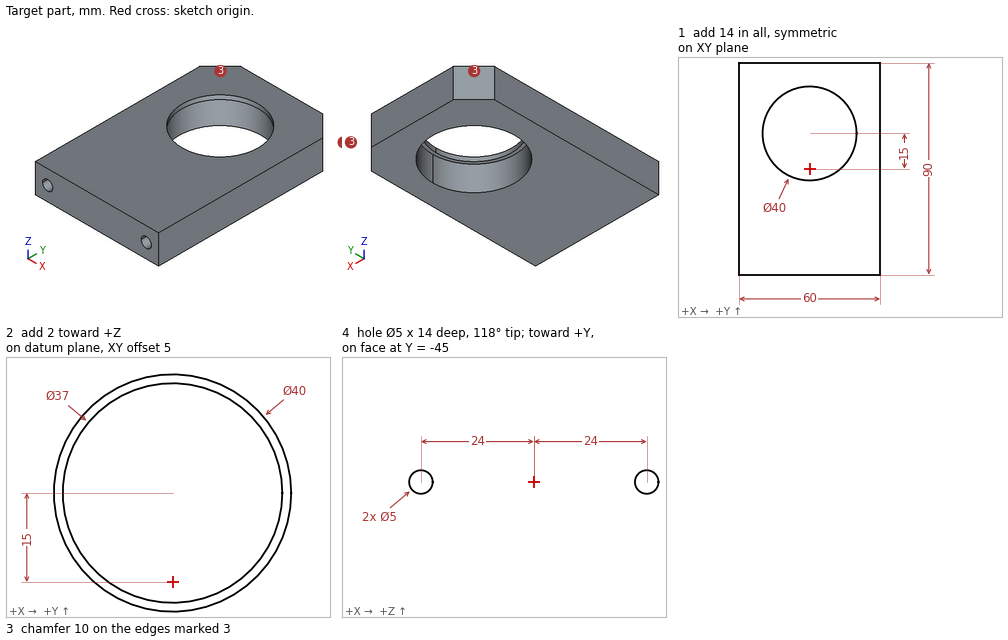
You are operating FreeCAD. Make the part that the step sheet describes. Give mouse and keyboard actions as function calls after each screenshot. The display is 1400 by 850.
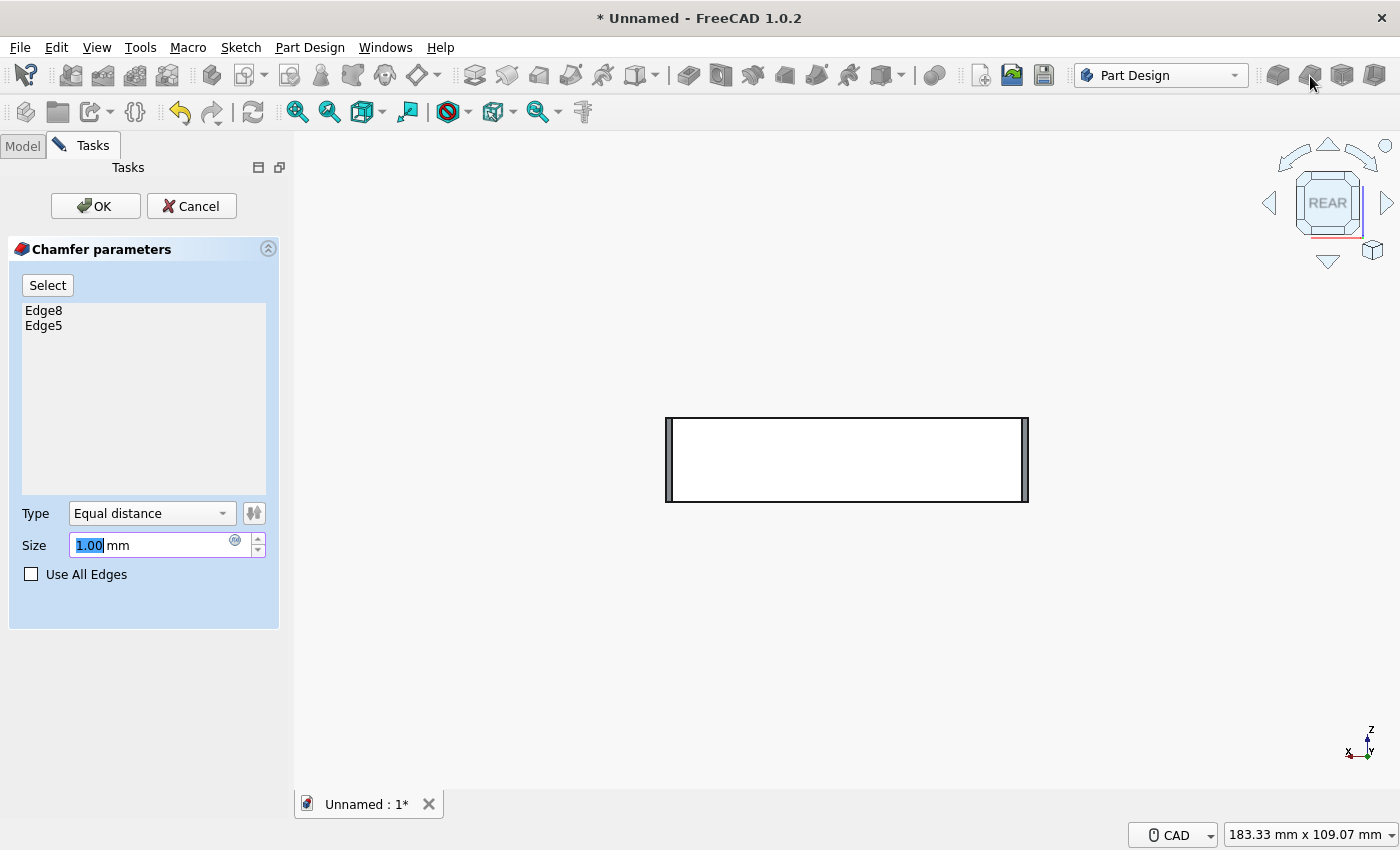
text(10)
key(Tab)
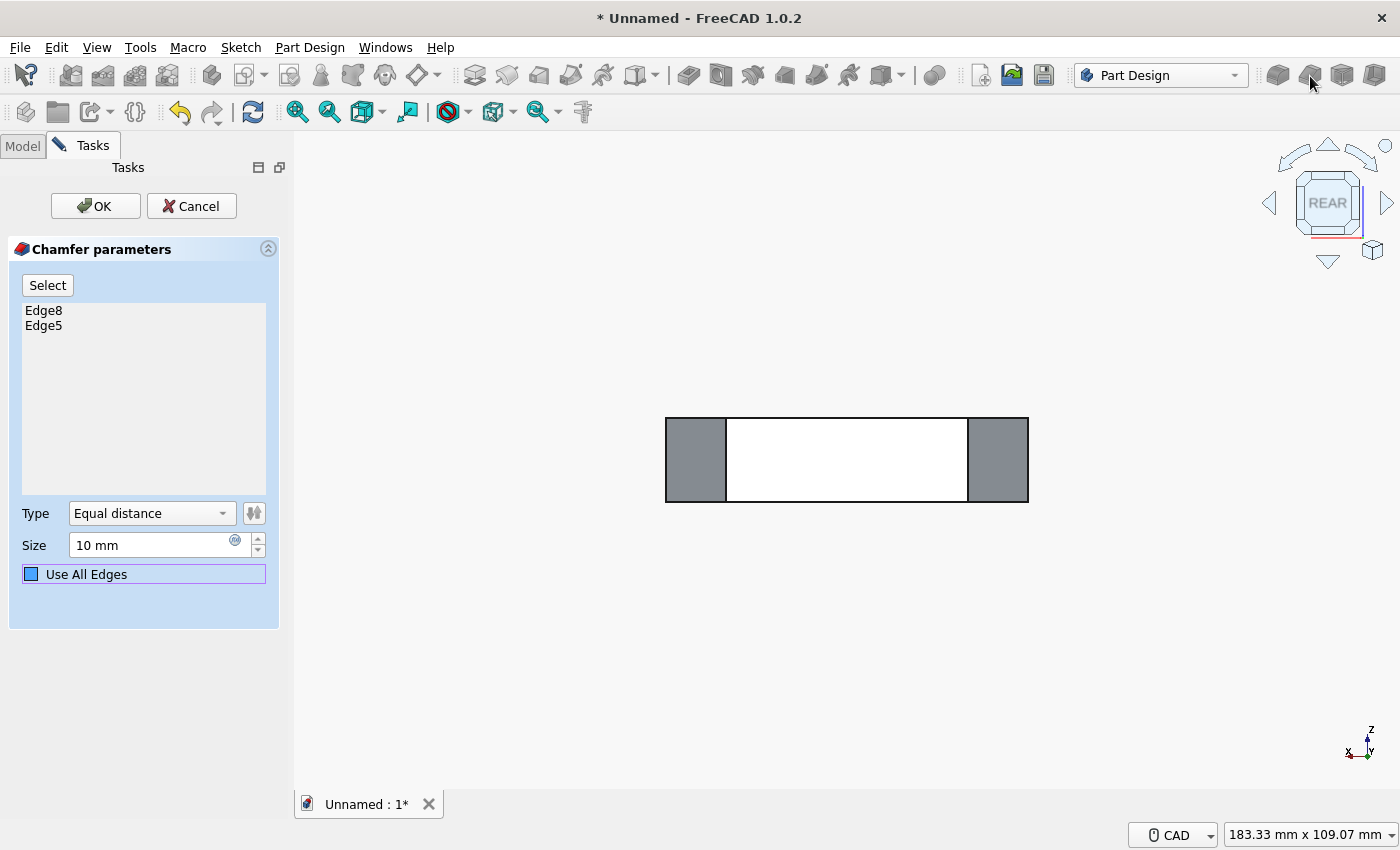
click(96, 206)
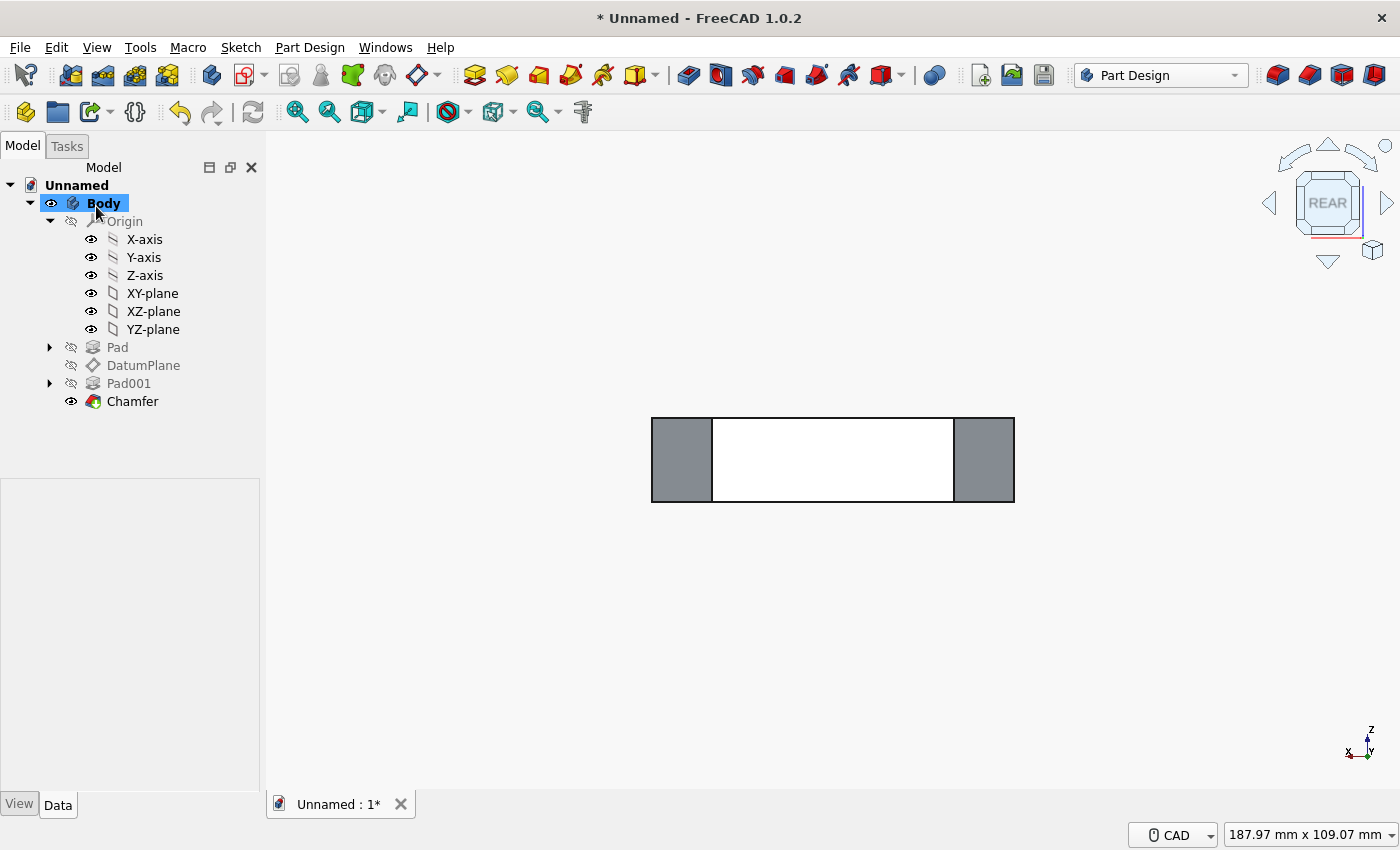
click(298, 112)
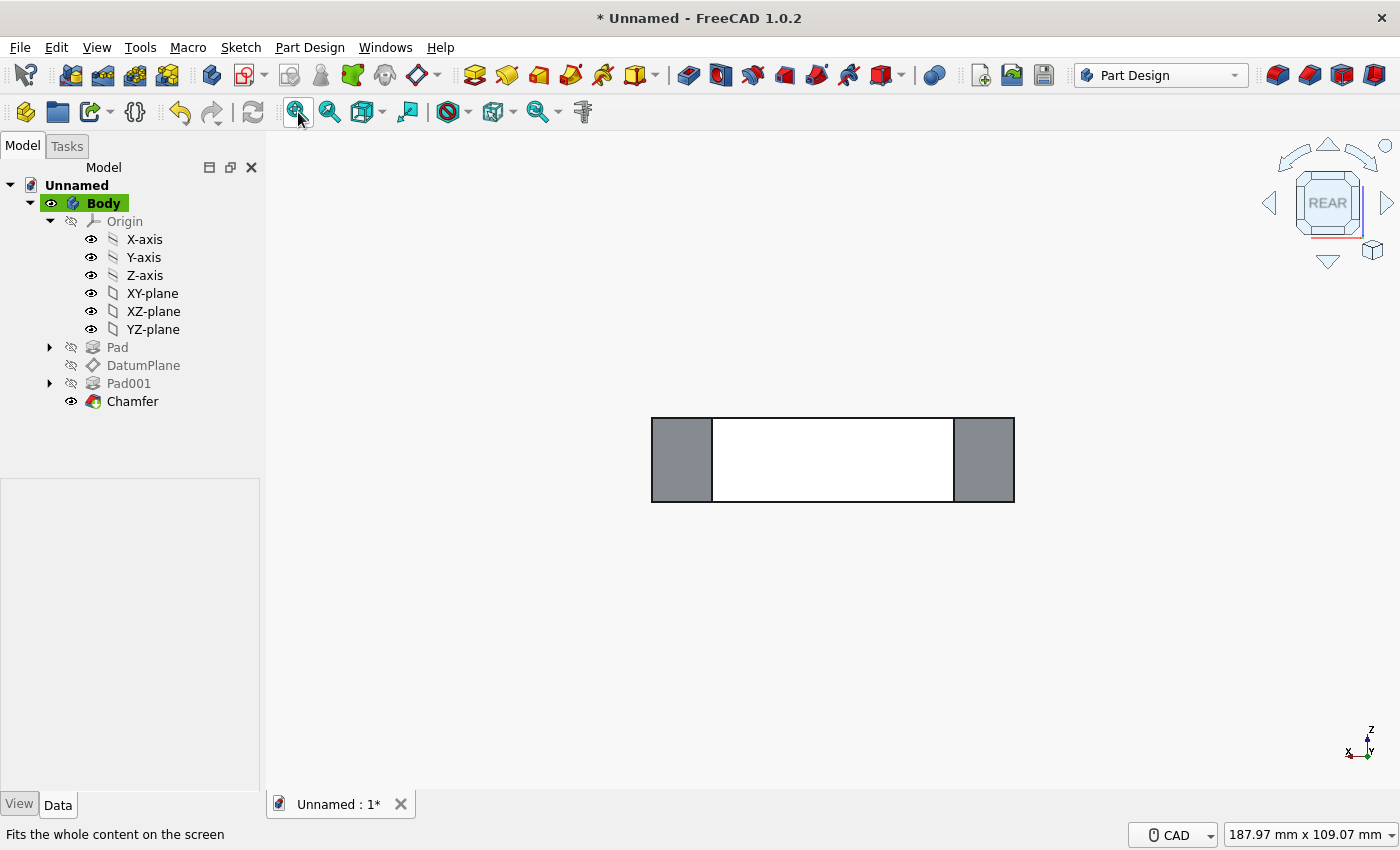
key(0)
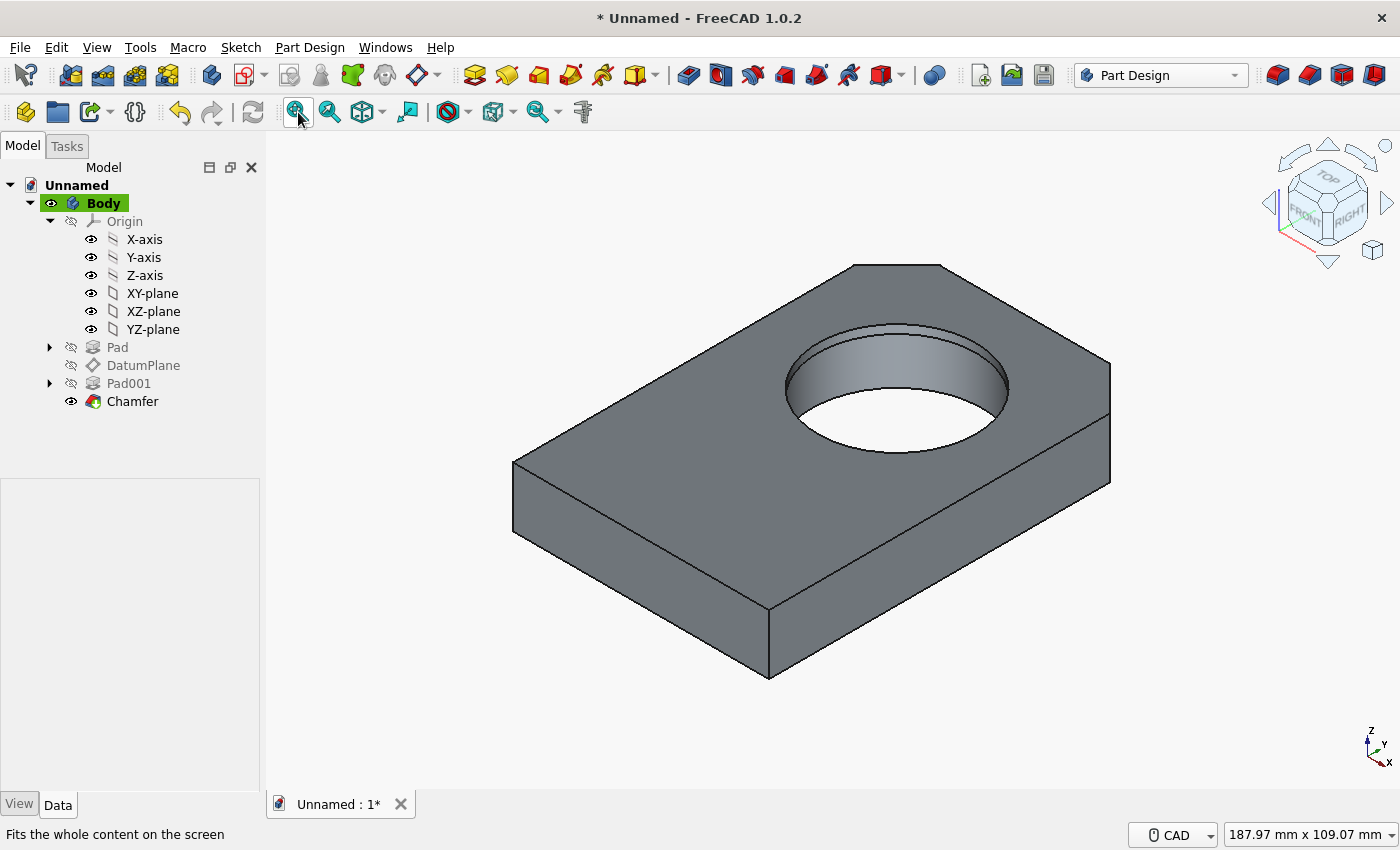
click(714, 612)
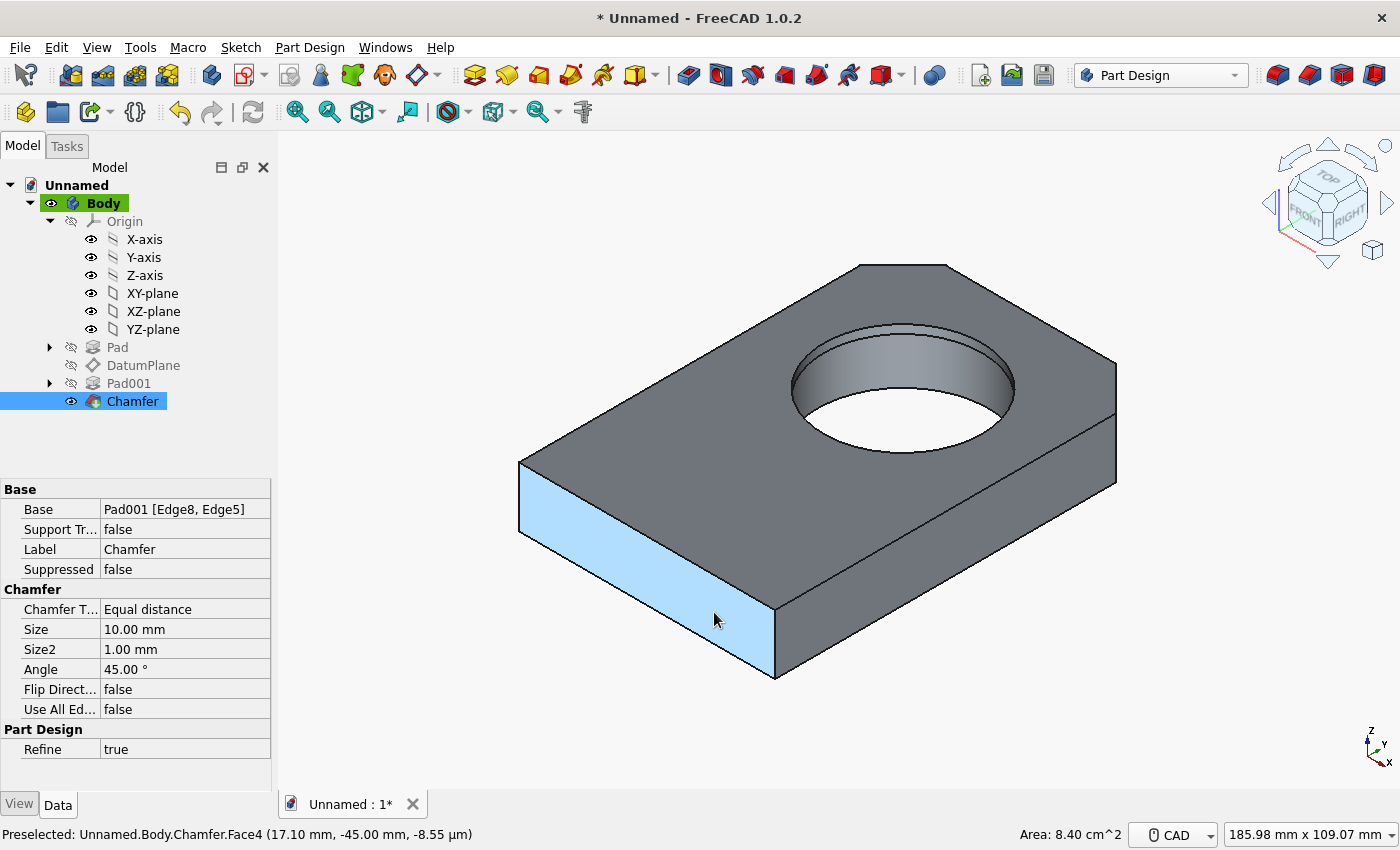
click(244, 76)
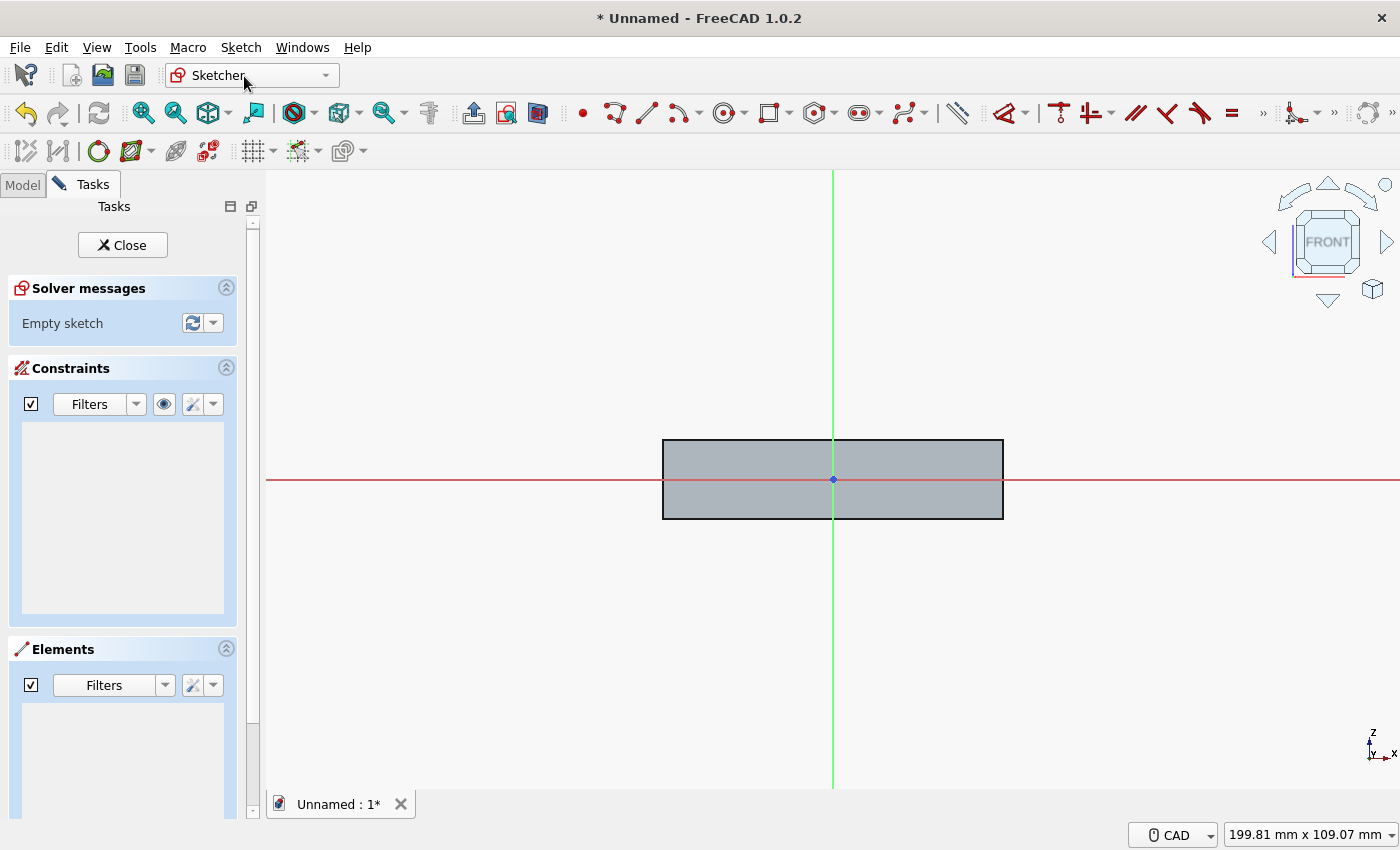
scroll(889, 480, up, 4)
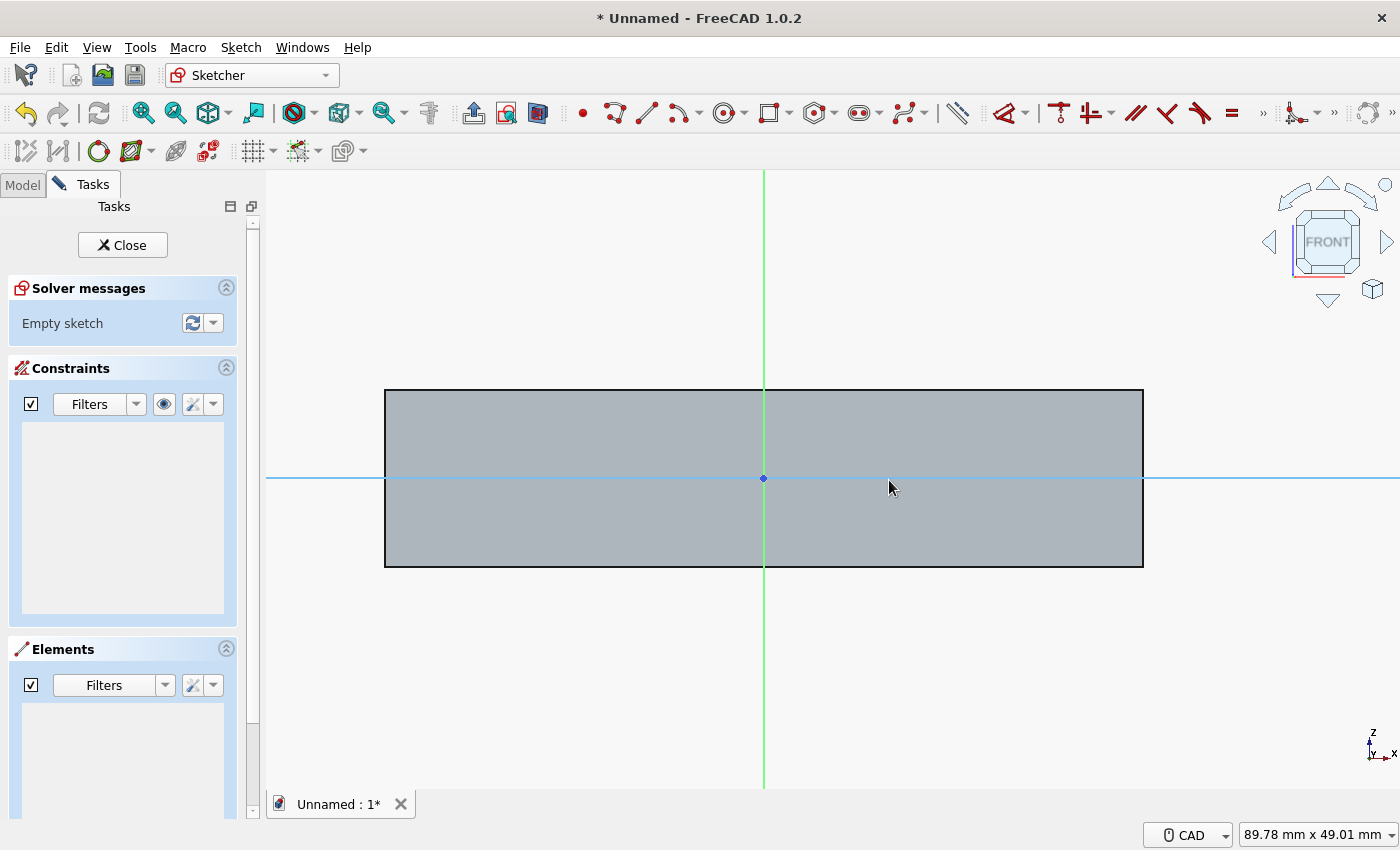
click(724, 114)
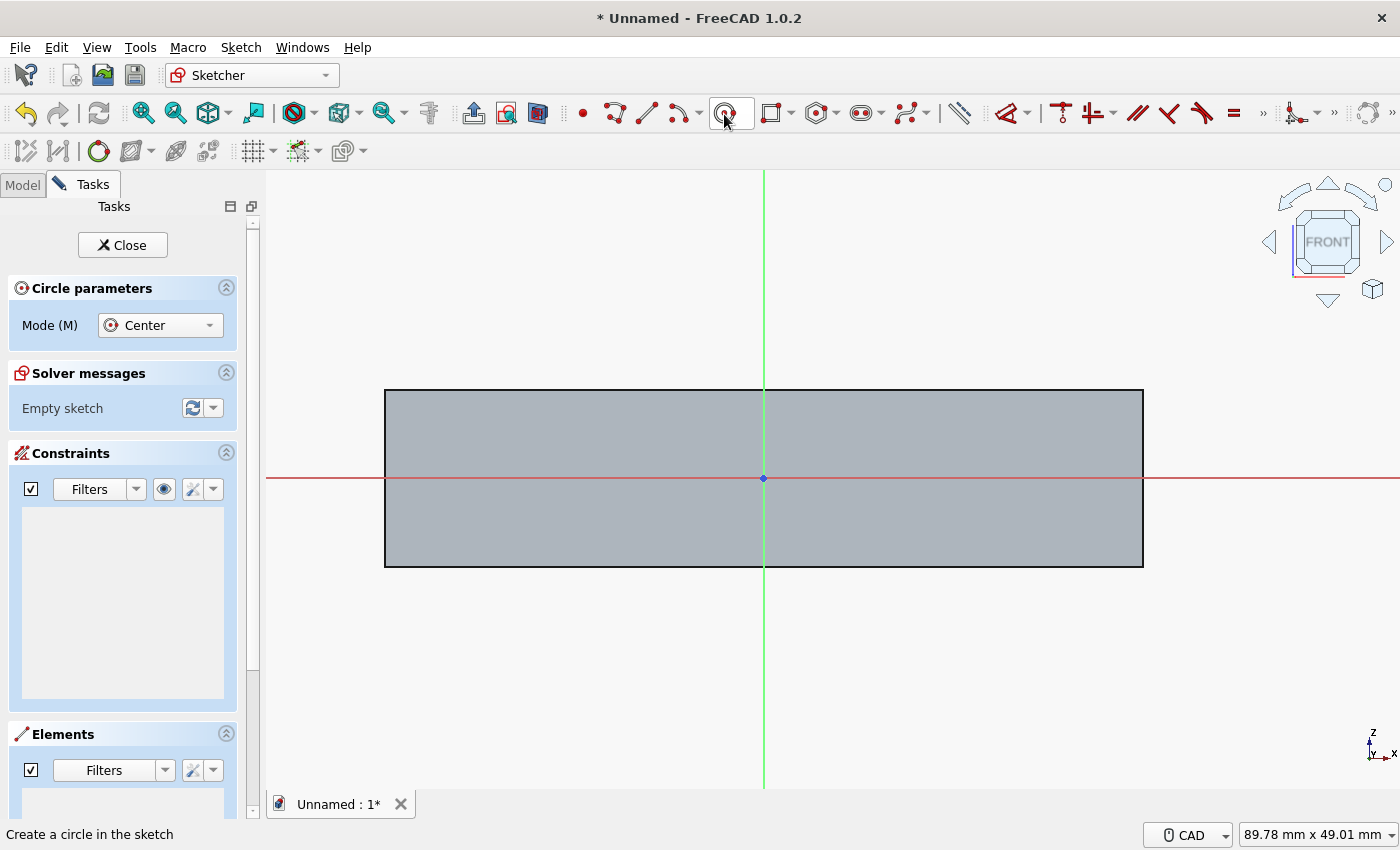
click(461, 478)
move(483, 456)